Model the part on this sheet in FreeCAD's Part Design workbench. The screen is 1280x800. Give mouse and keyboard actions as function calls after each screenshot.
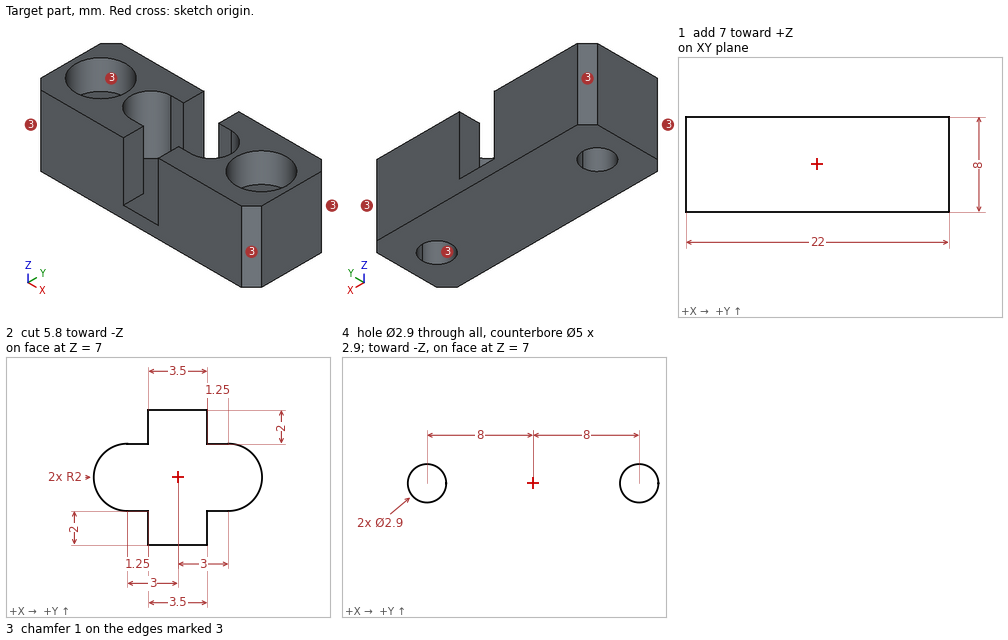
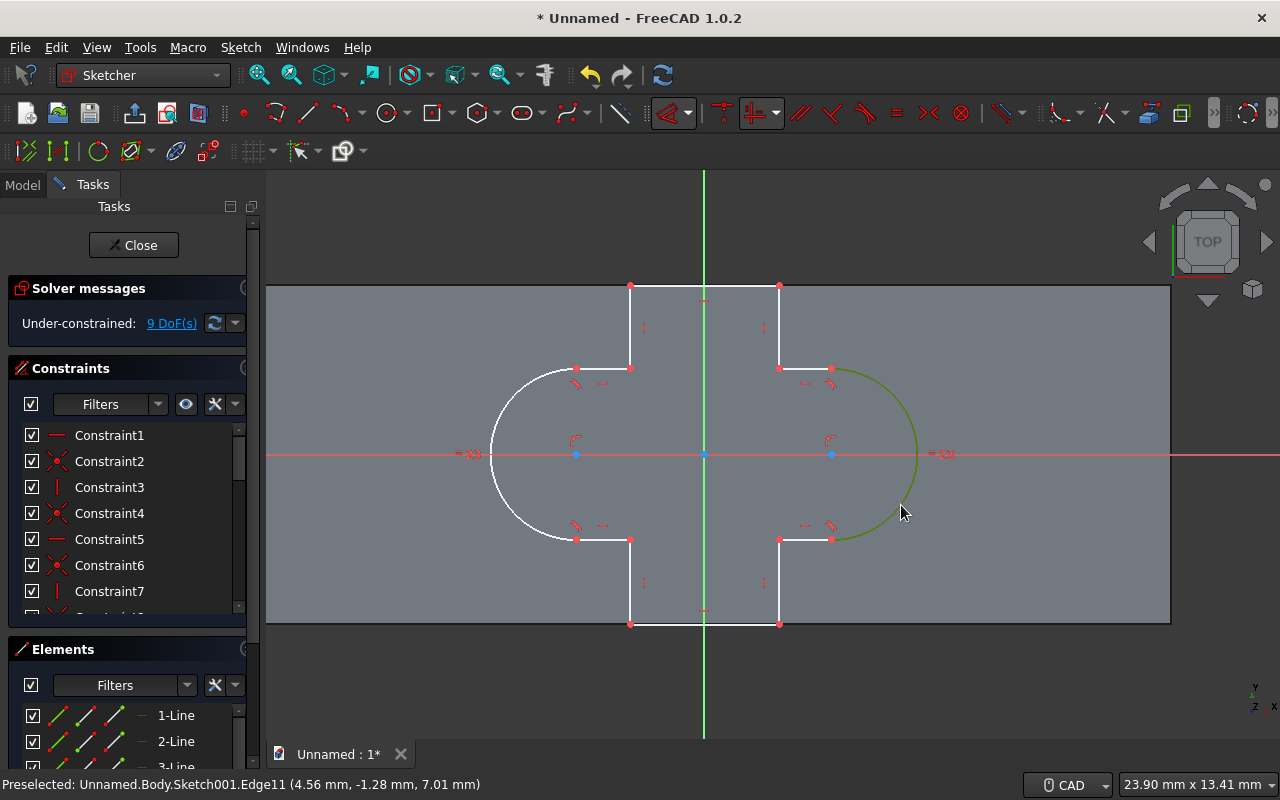
key(k)
key(r)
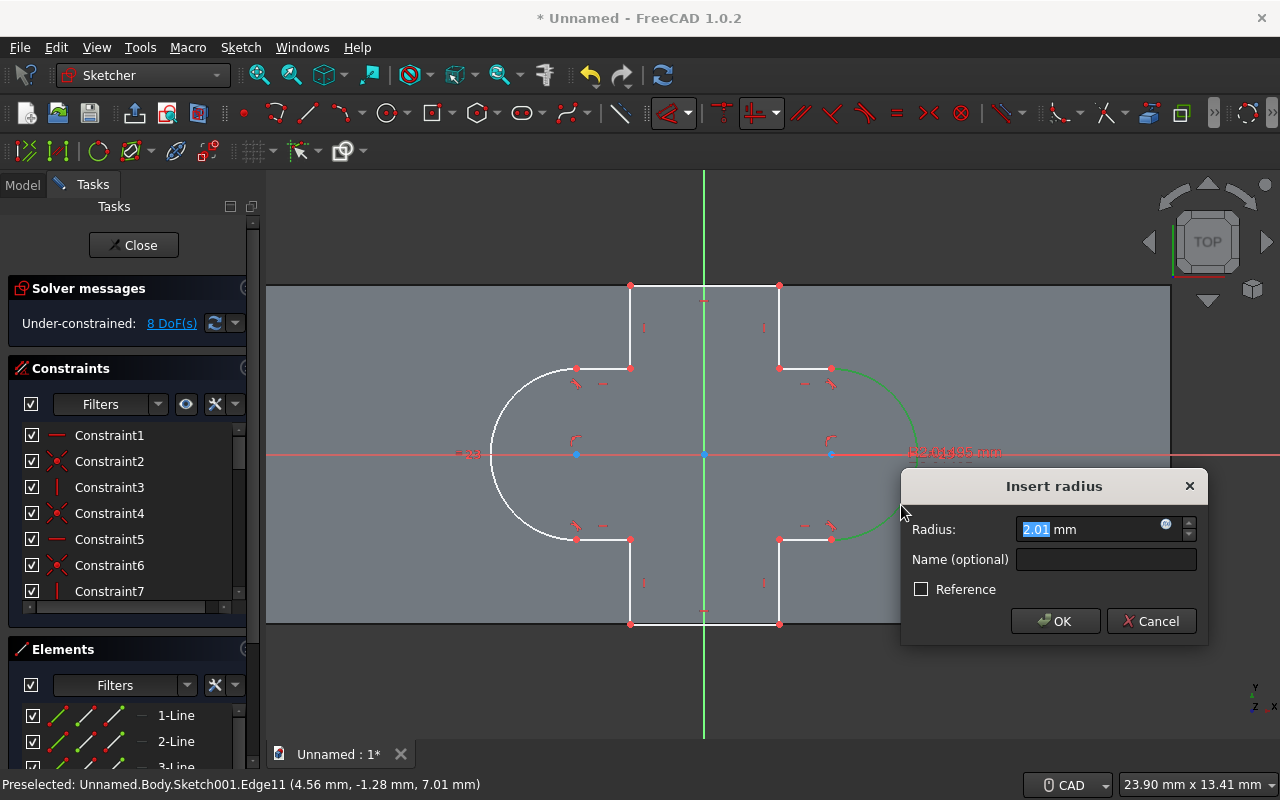
text(2)
key(Return)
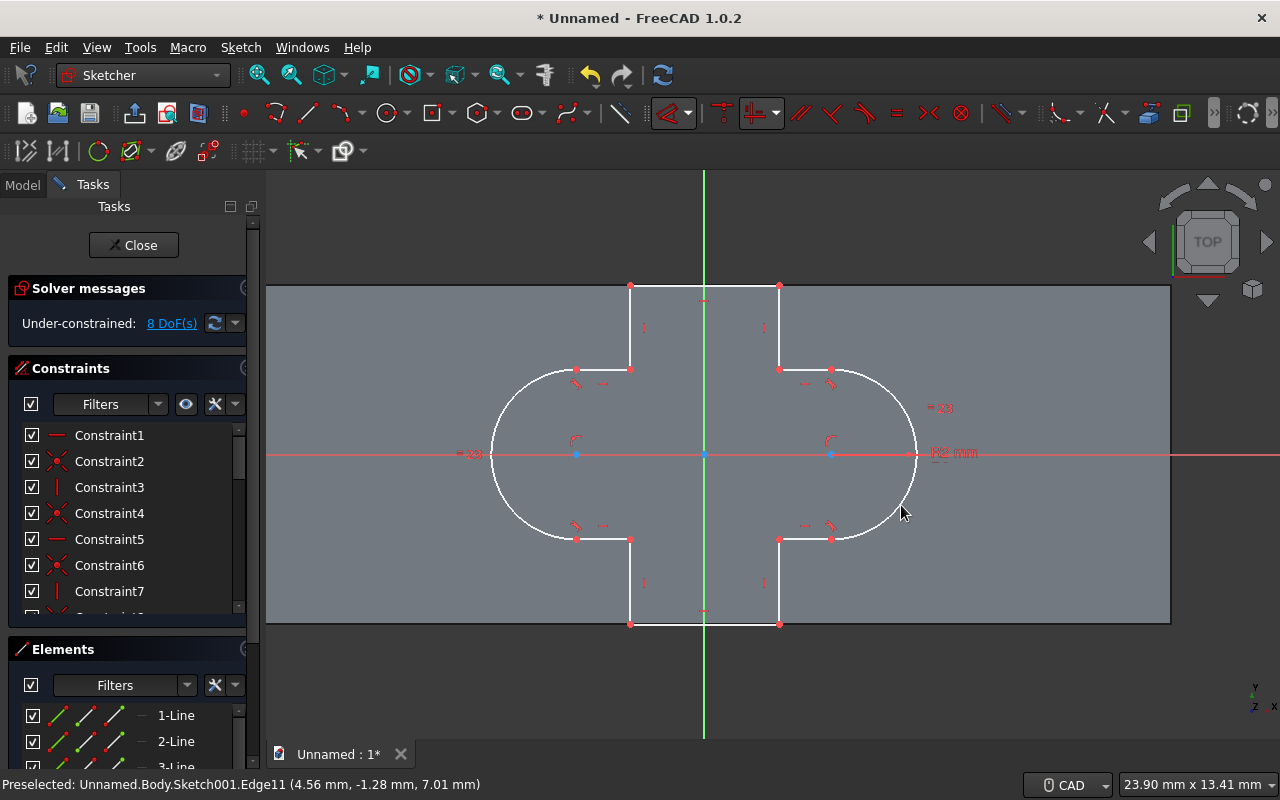
click(630, 565)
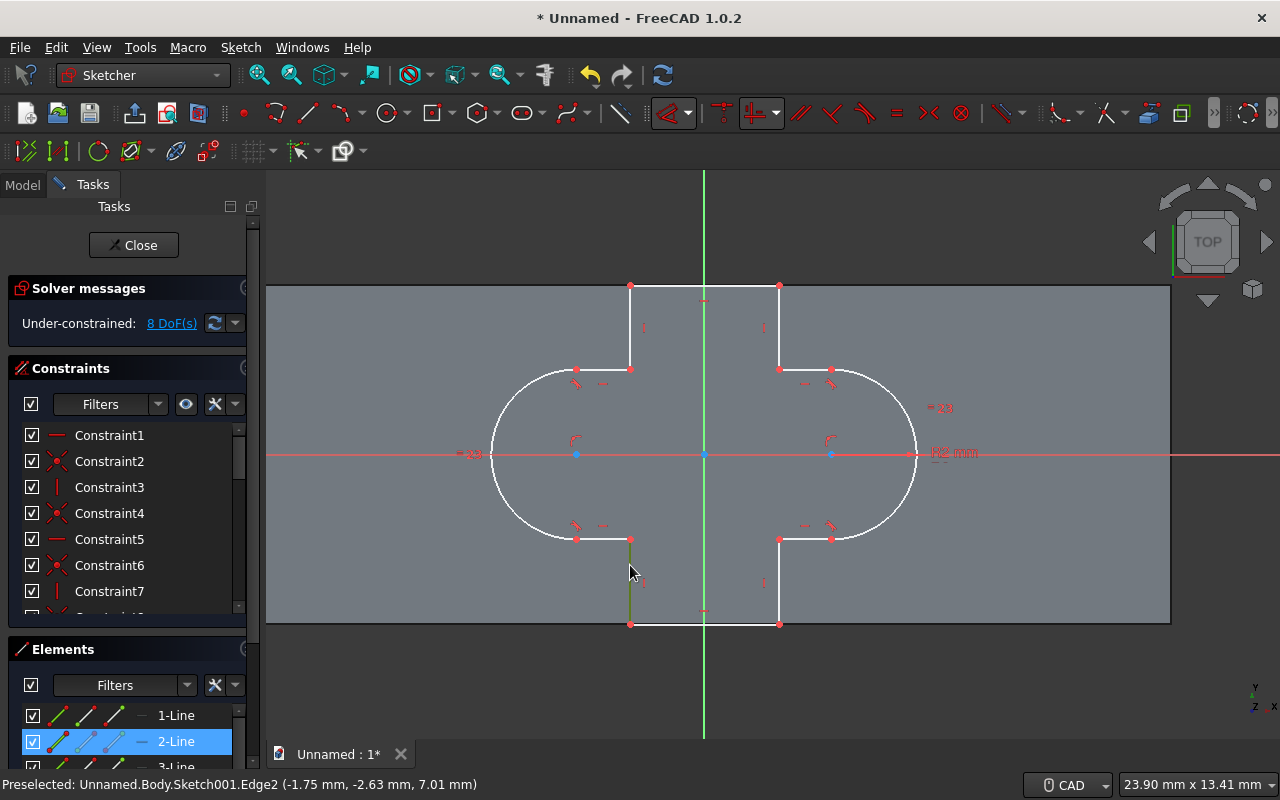
key(i)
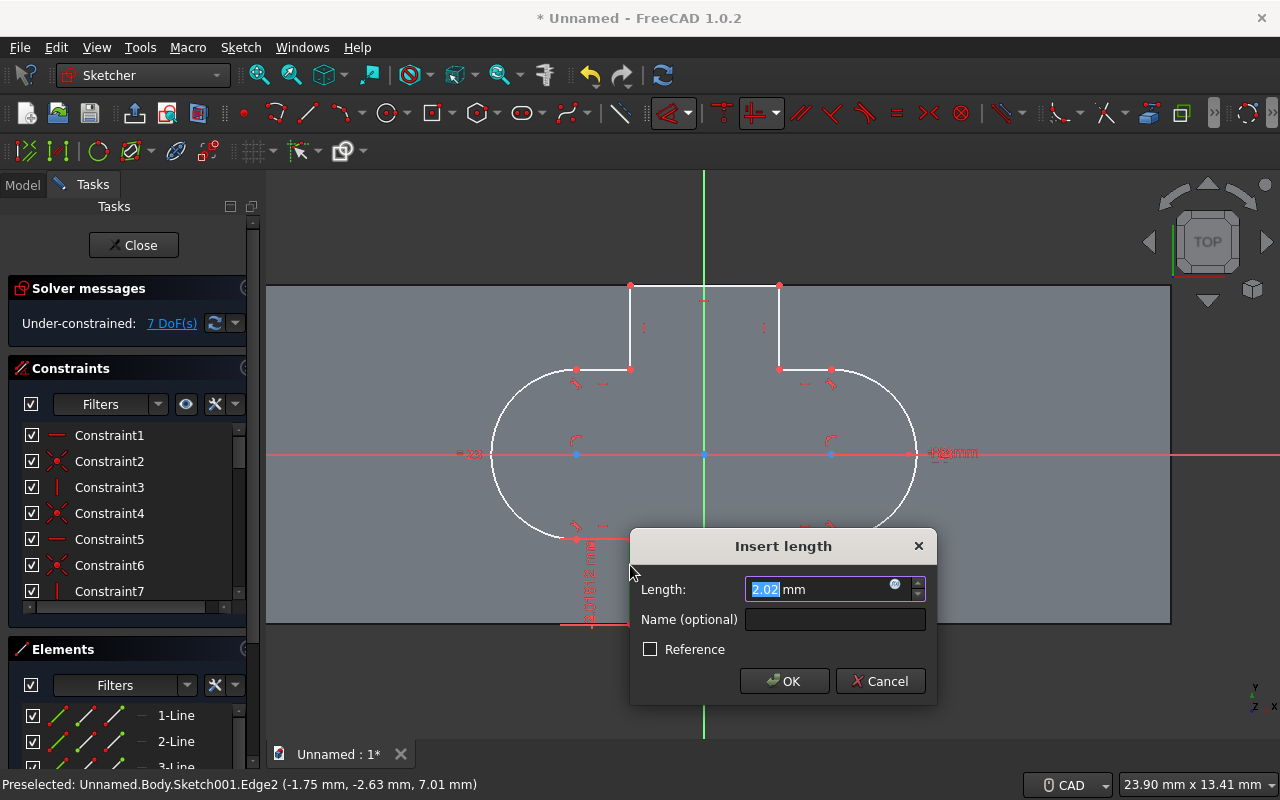
text(2)
key(Return)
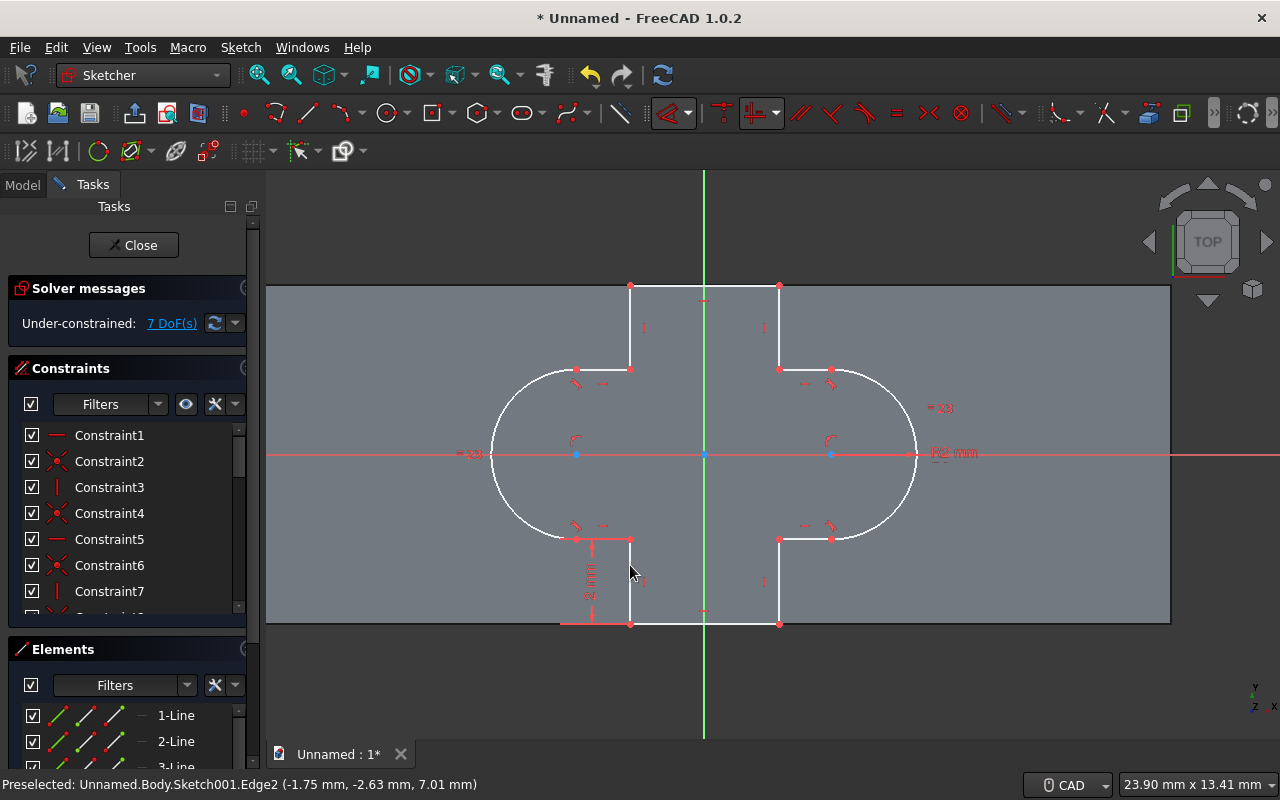
click(779, 345)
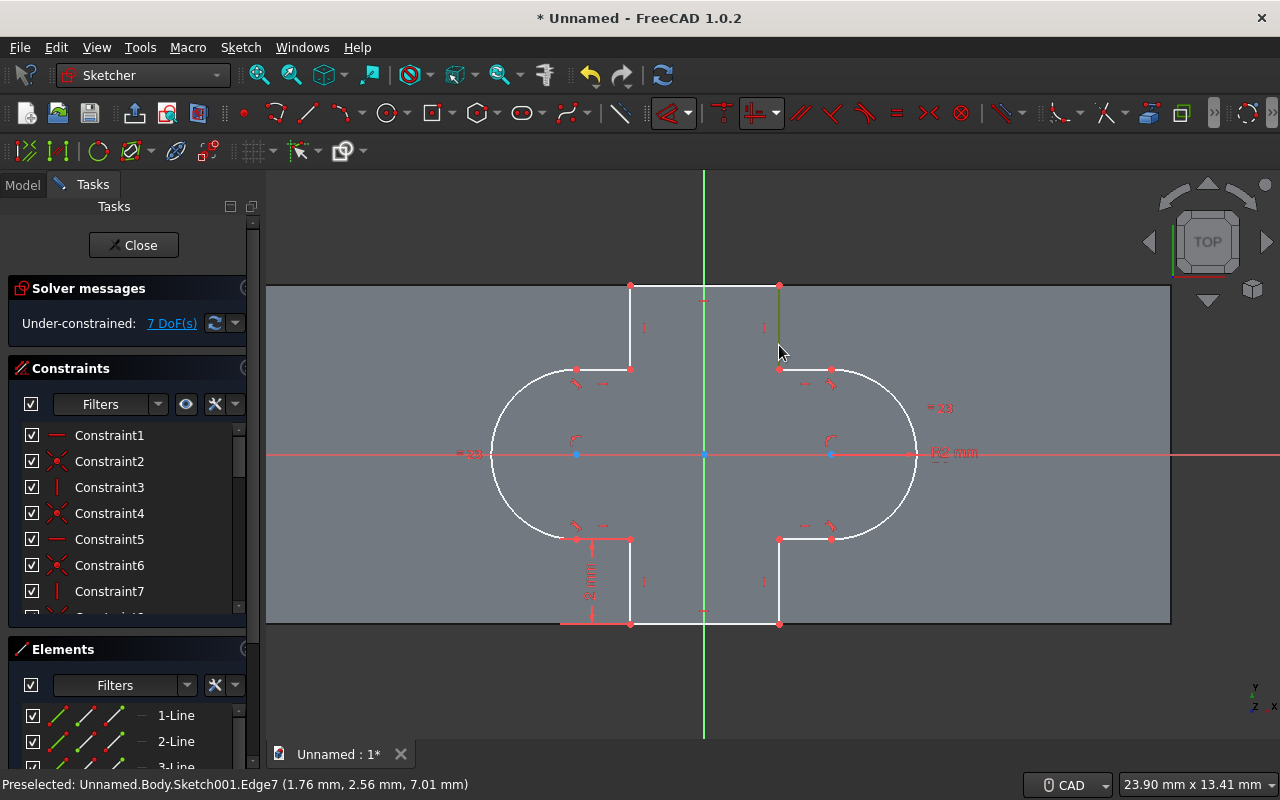
key(i)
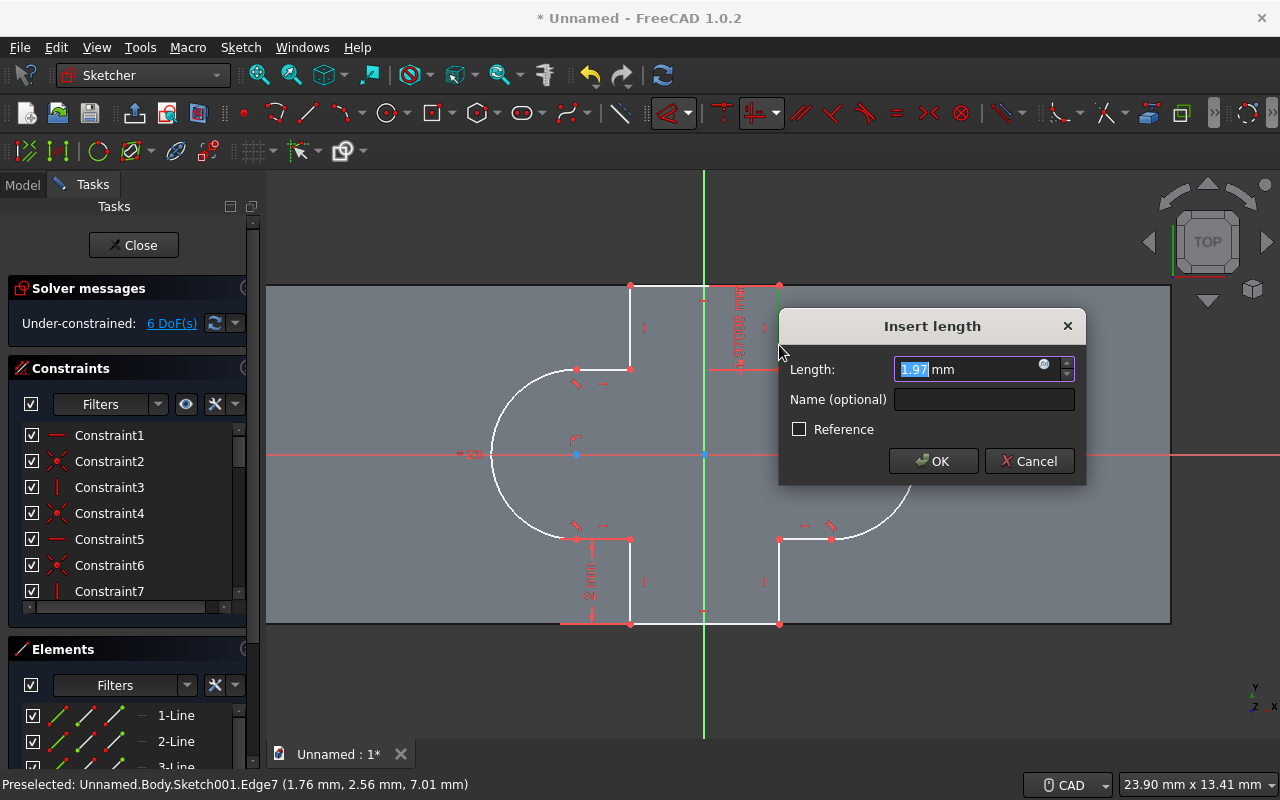
text(2)
key(Return)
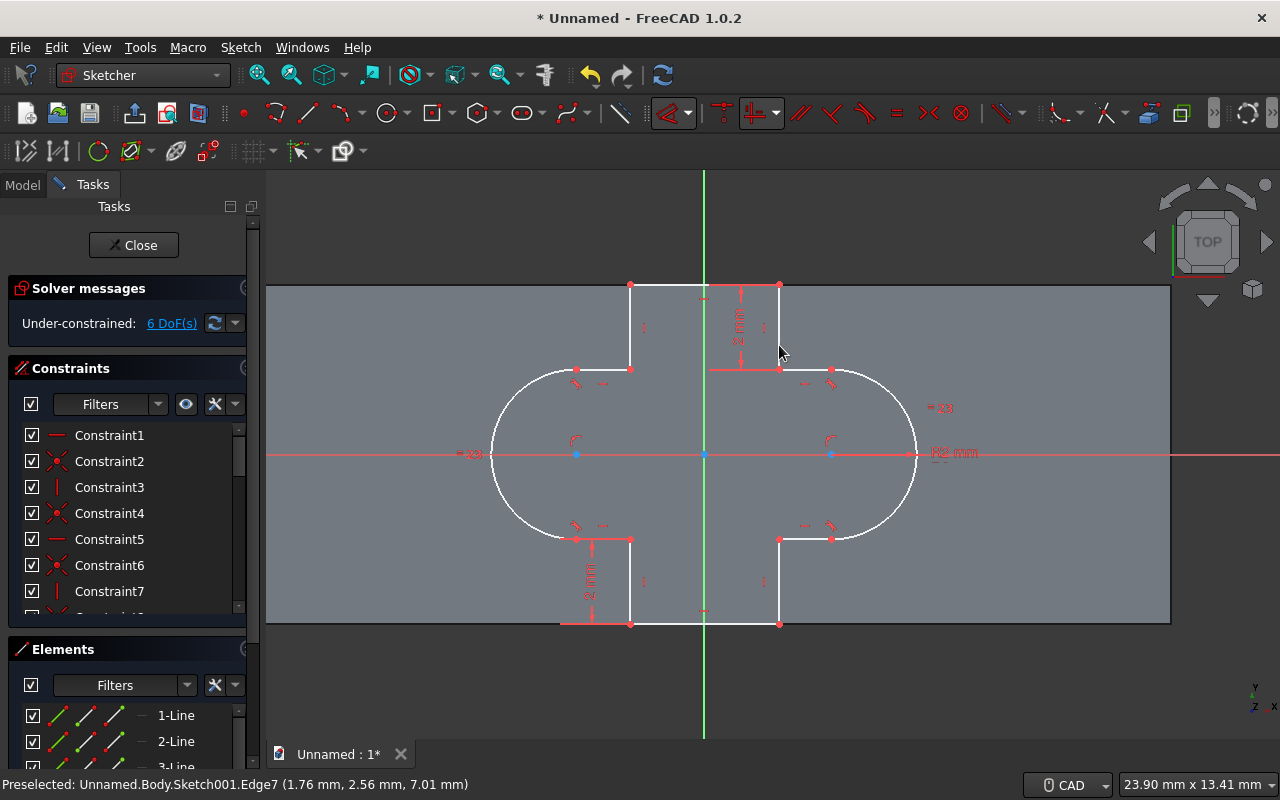
click(576, 539)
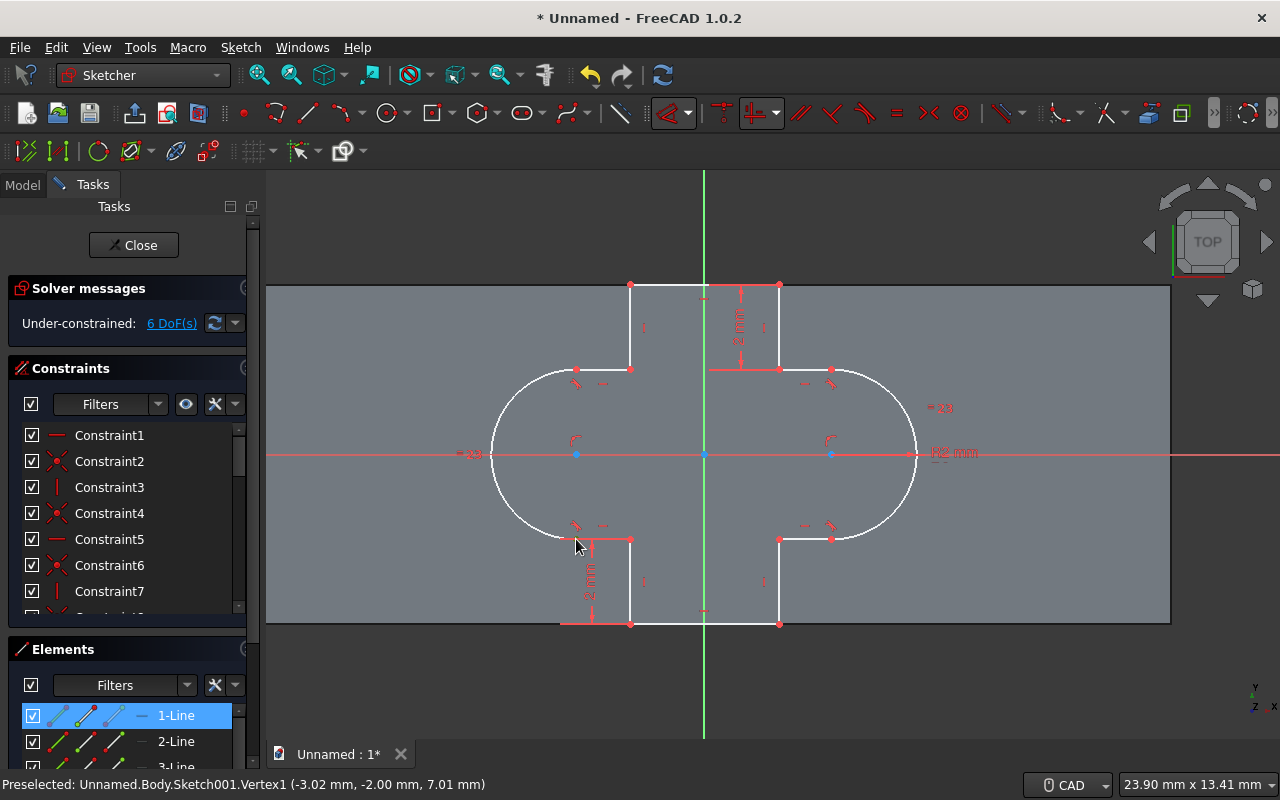
click(690, 114)